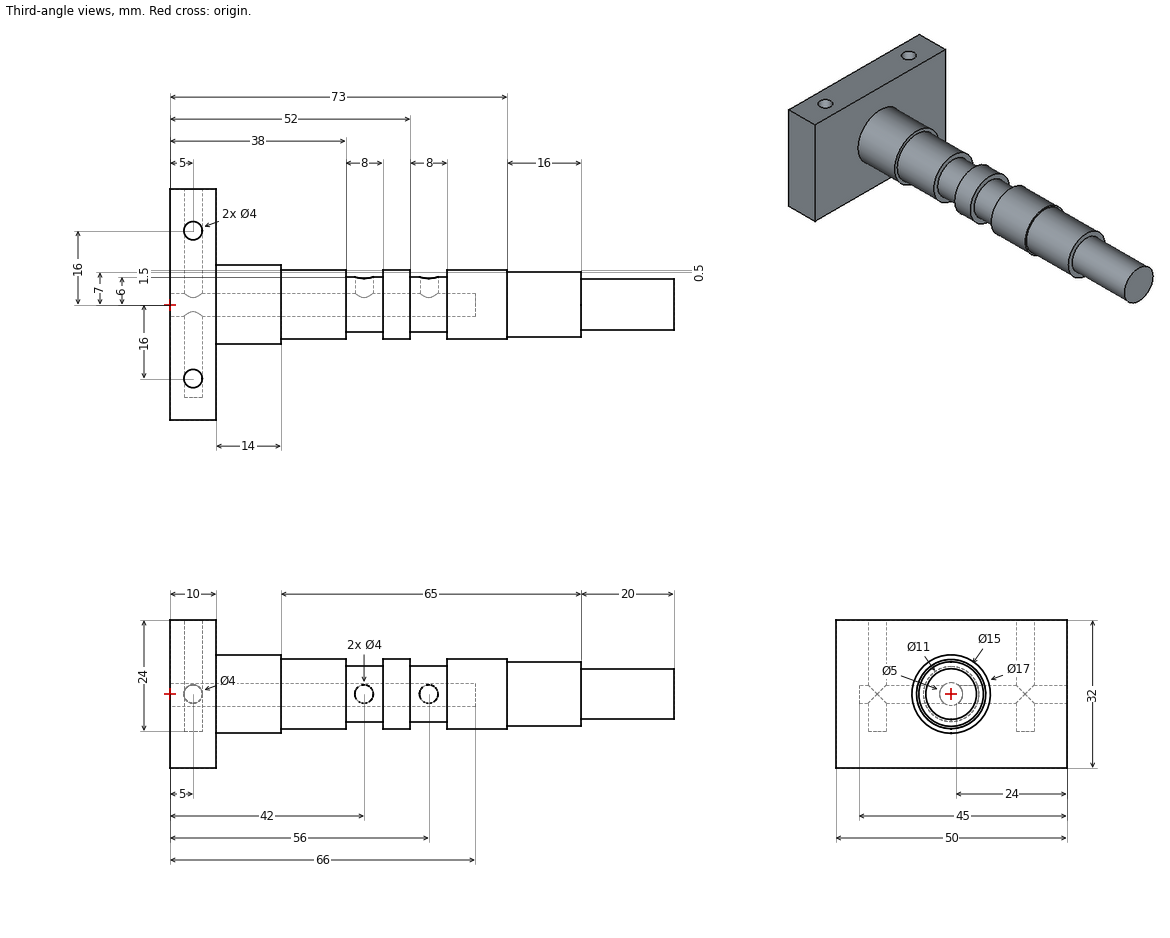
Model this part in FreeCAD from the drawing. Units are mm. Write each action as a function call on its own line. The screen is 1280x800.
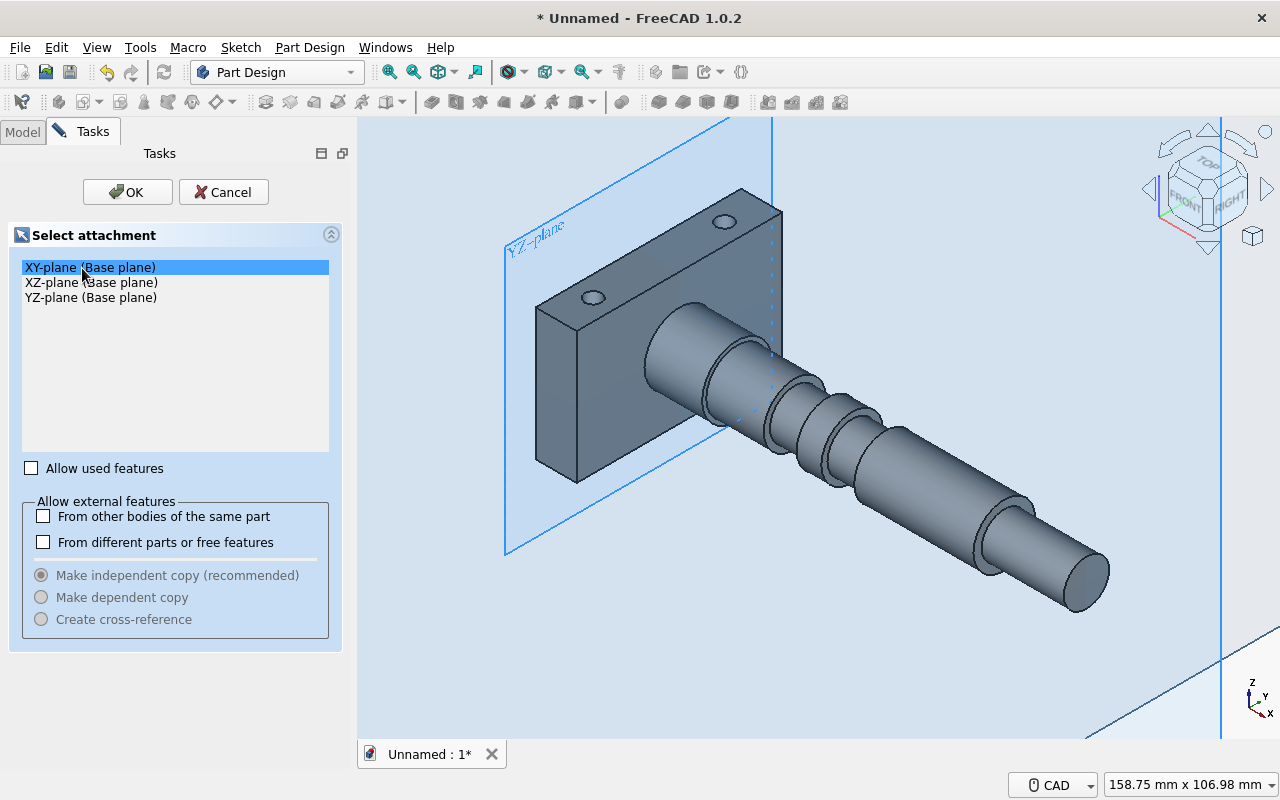
click(128, 192)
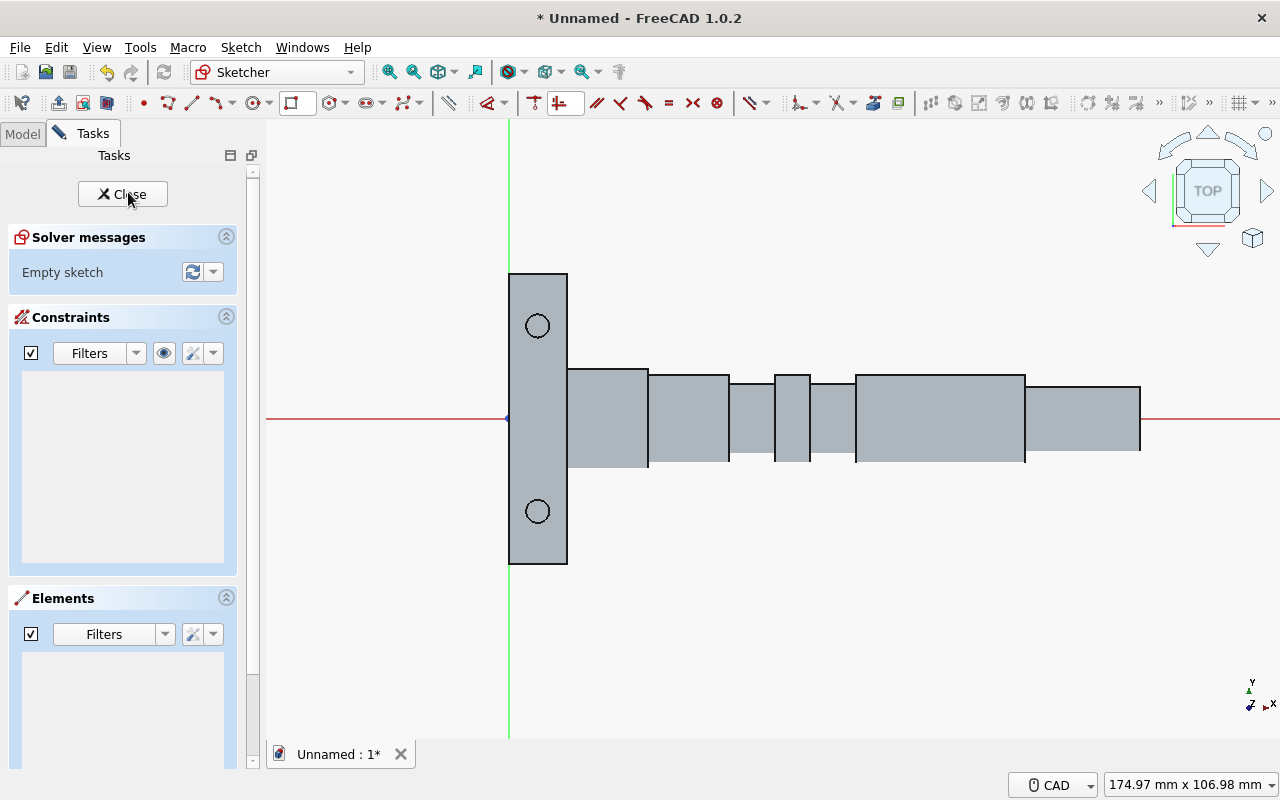
click(108, 104)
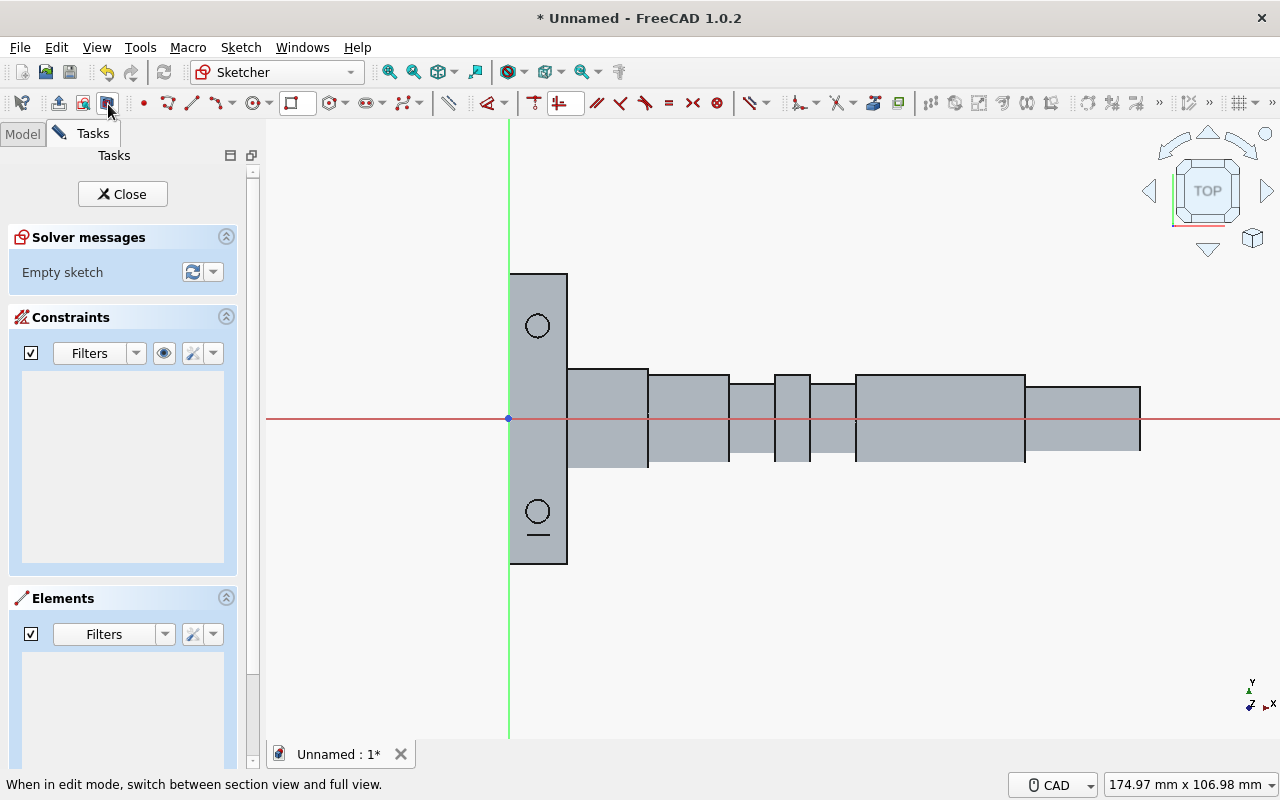
scroll(1032, 366, up, 9)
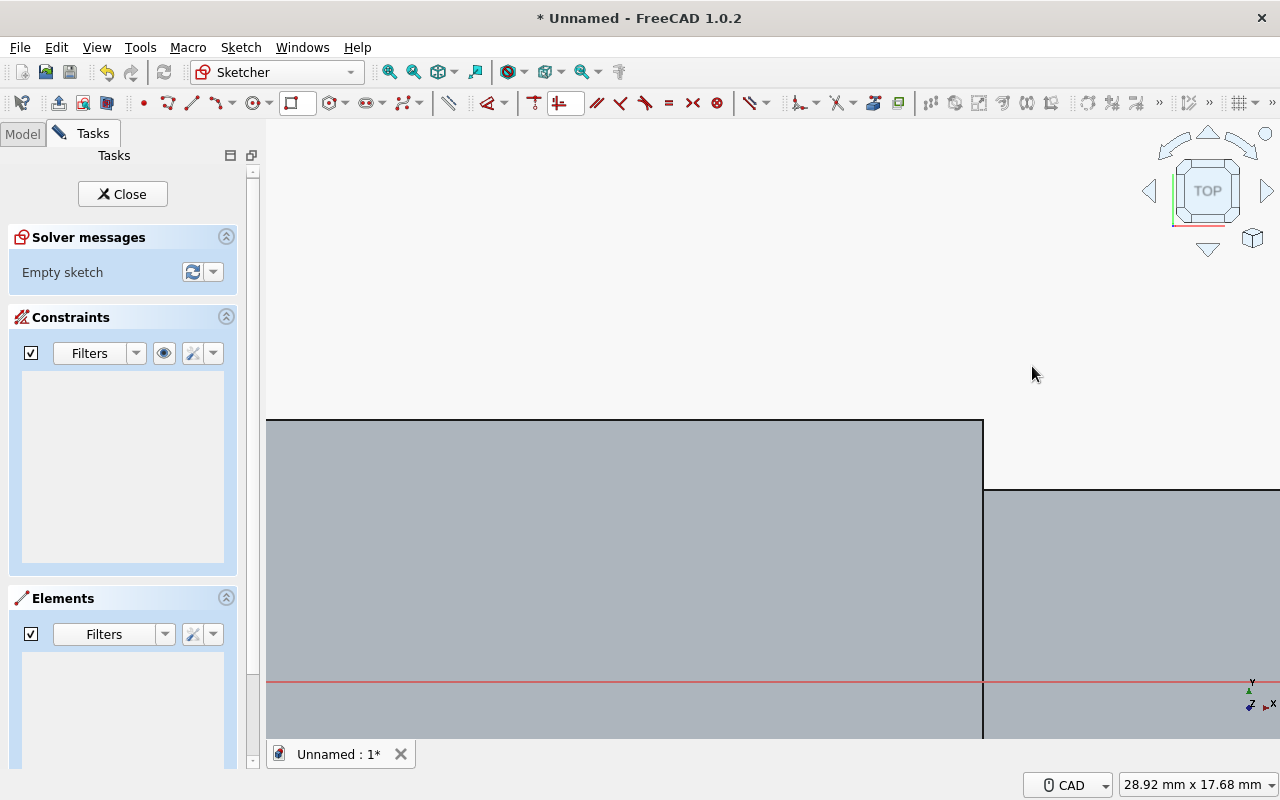
click(292, 104)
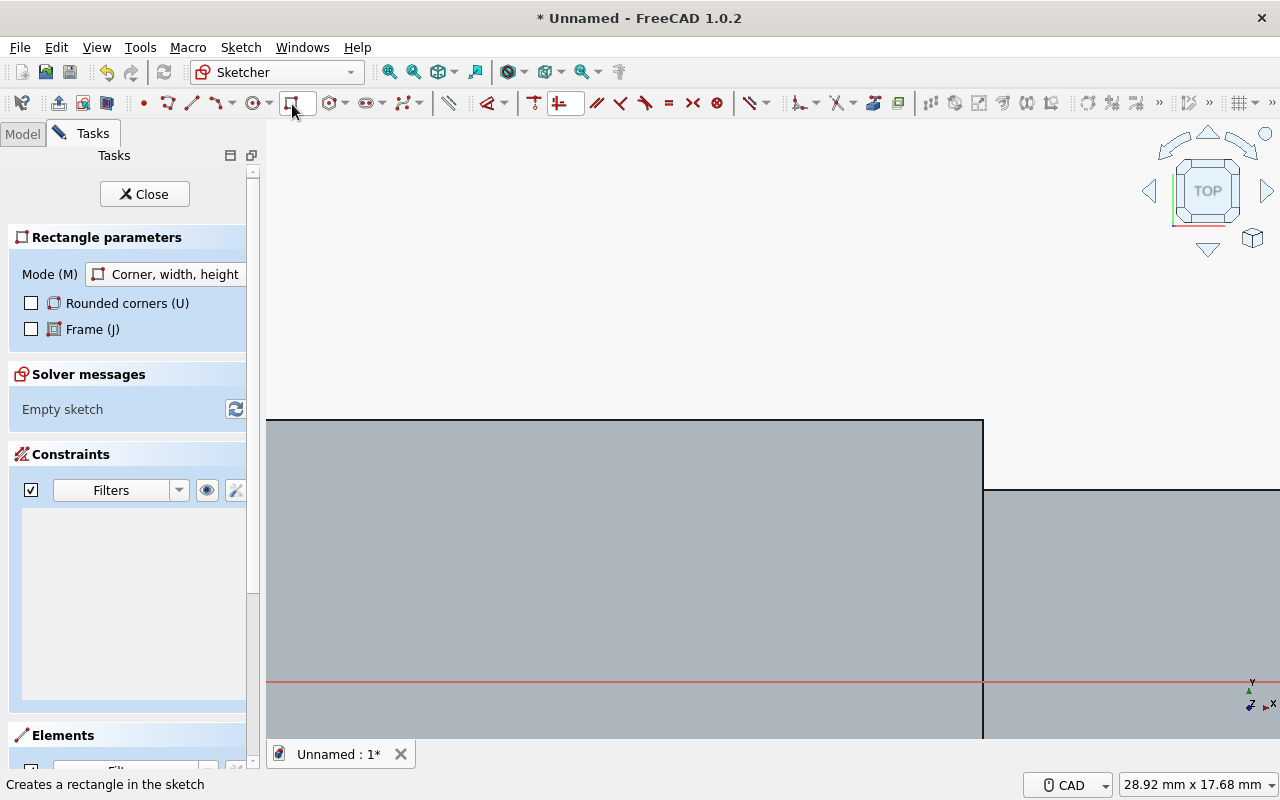
click(422, 420)
move(983, 437)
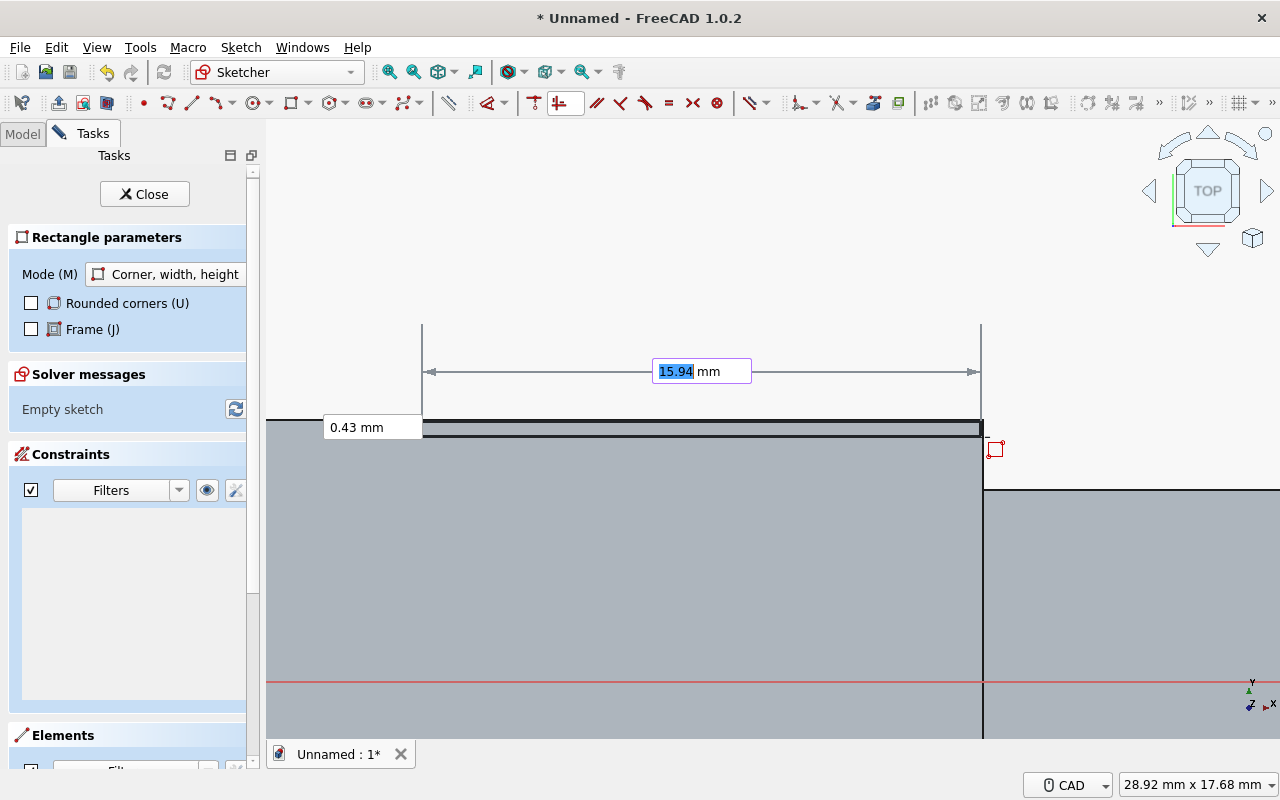
text(16)
key(Tab)
text(0.5)
key(Return)
key(Escape)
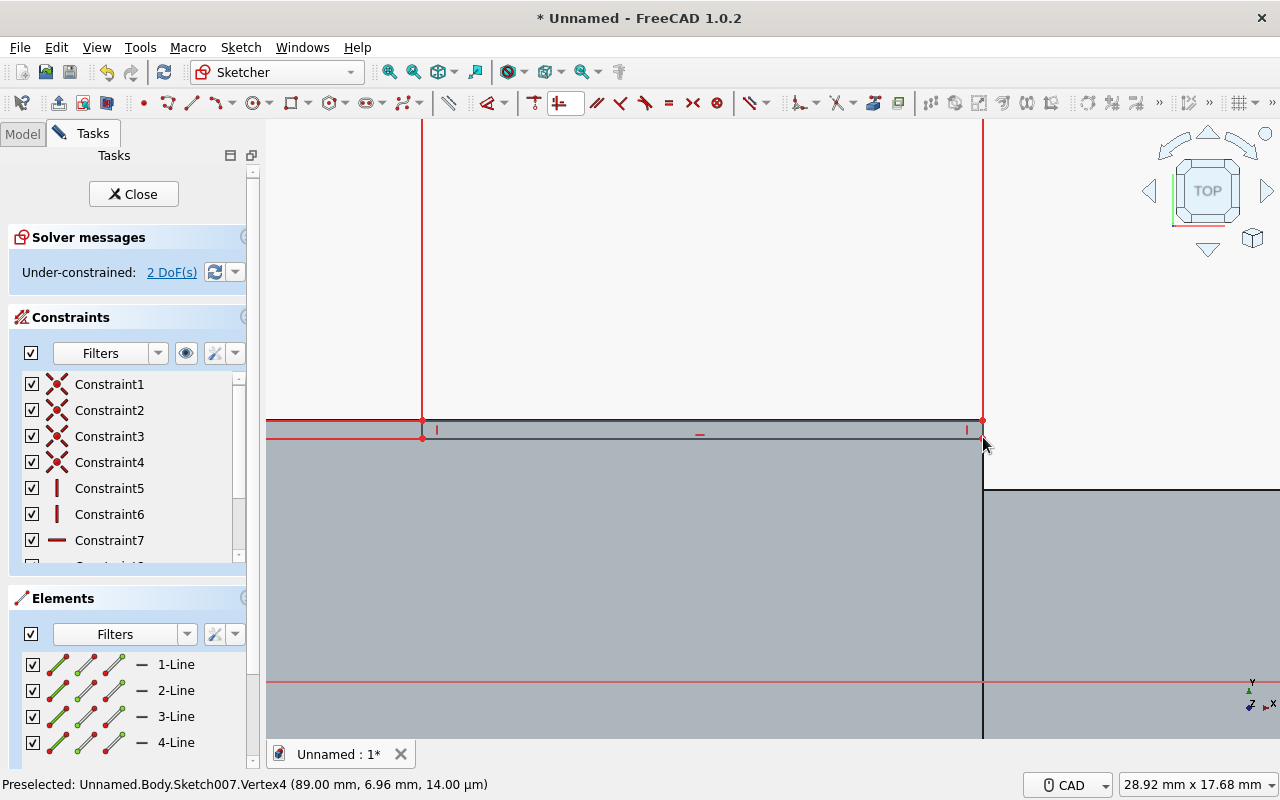
click(488, 104)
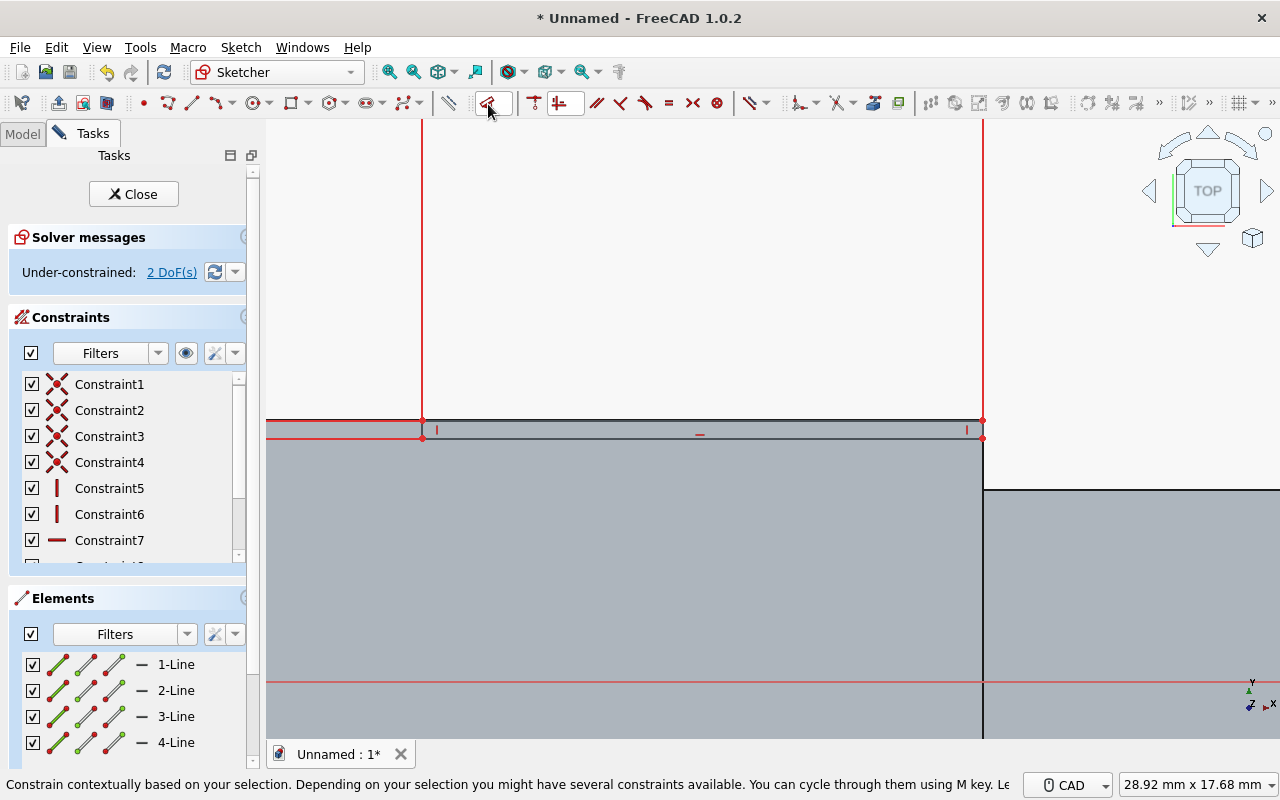
click(422, 439)
click(456, 560)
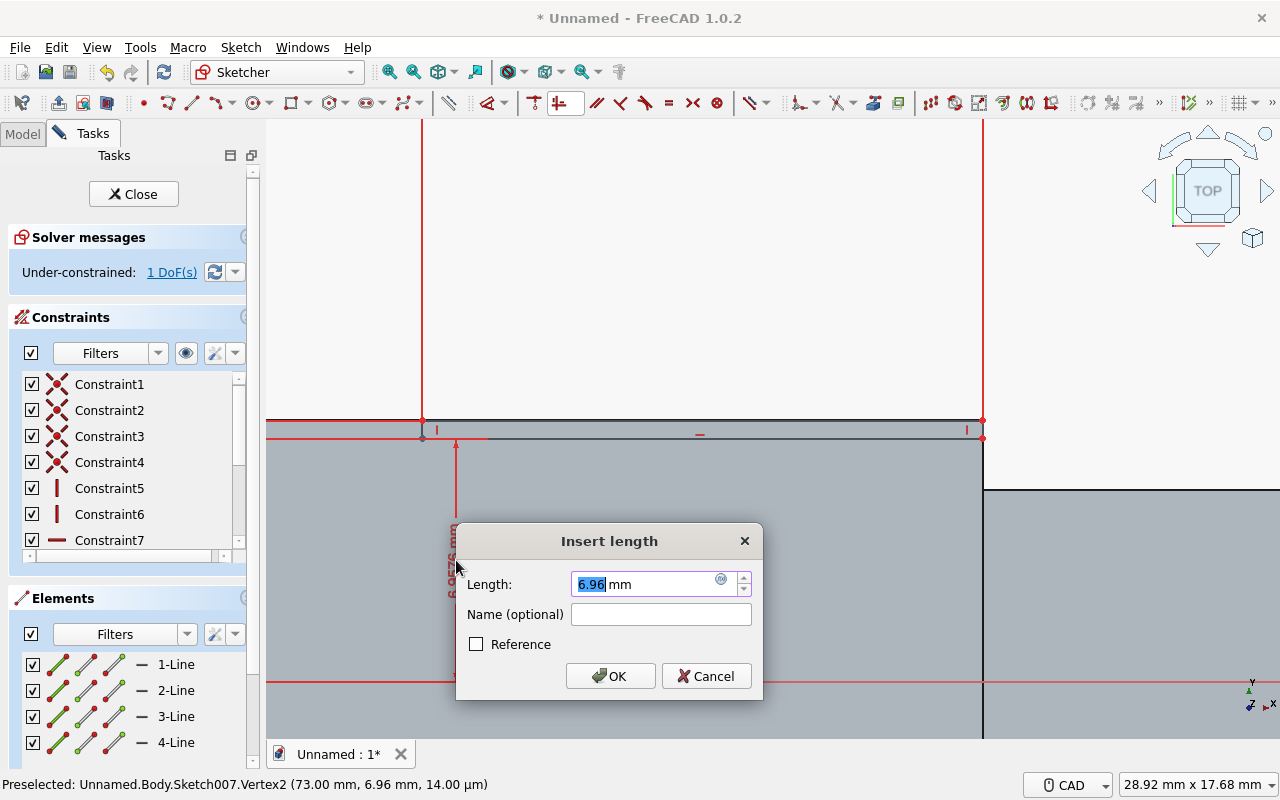
text(7)
key(Return)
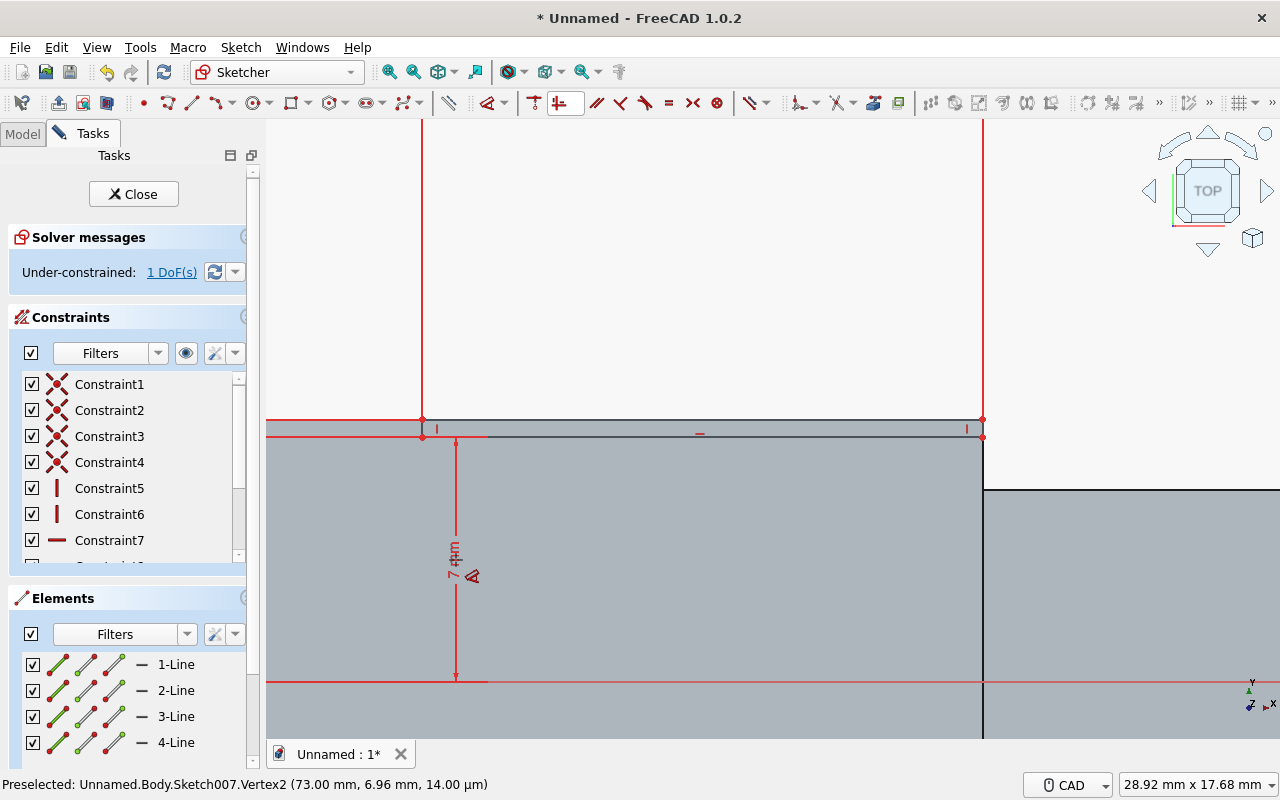
click(422, 420)
click(358, 386)